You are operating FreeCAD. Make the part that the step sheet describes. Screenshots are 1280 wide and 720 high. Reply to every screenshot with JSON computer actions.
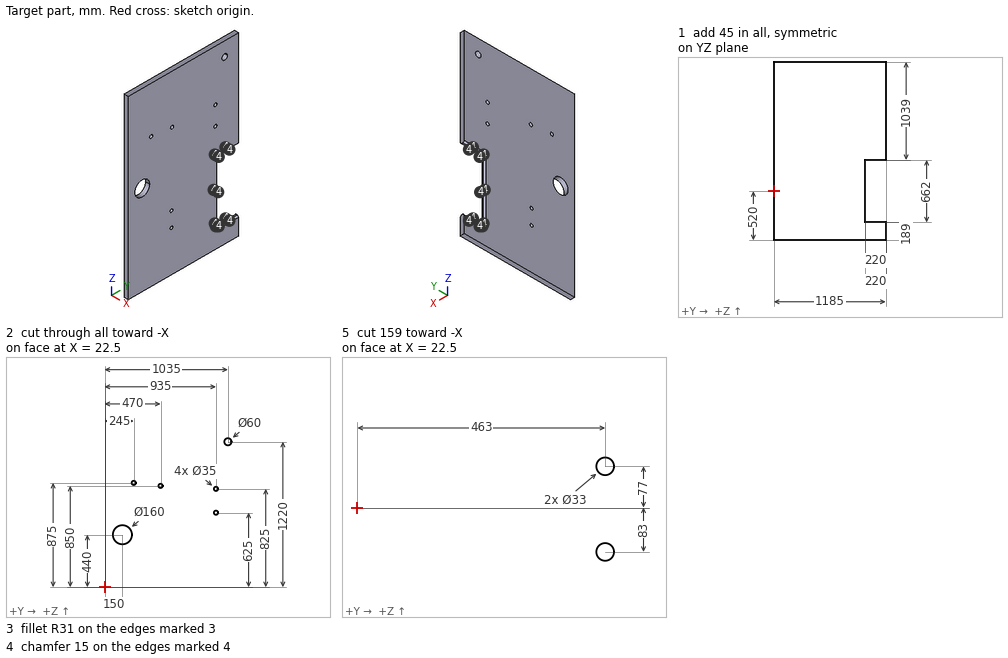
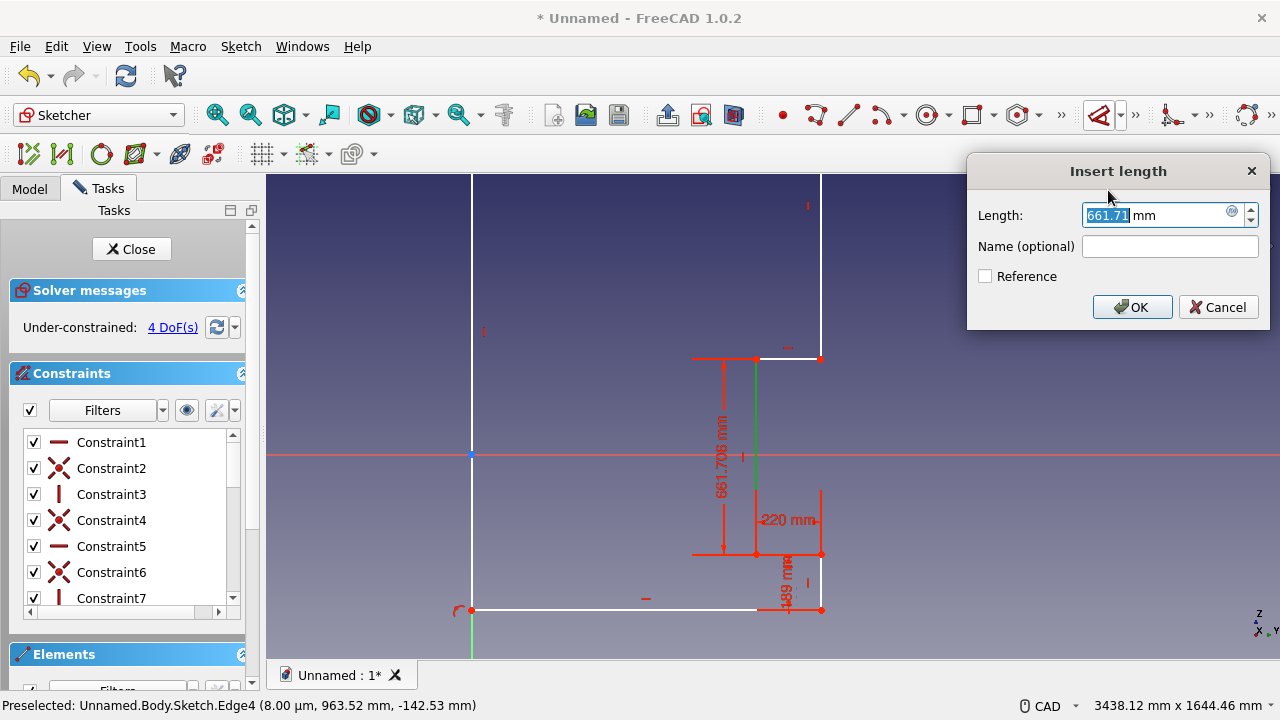
{"action": "type", "text": "662"}
{"action": "key", "text": "Return"}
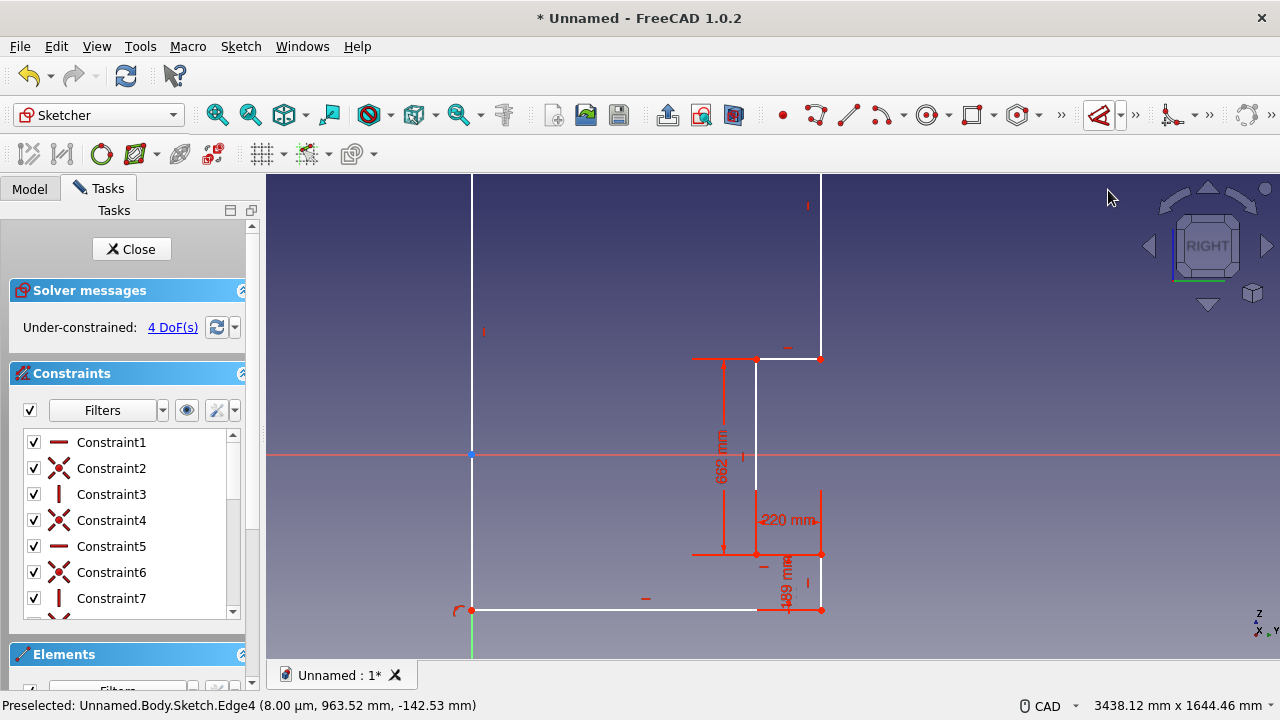
{"action": "left_click", "coordinate": [776, 359]}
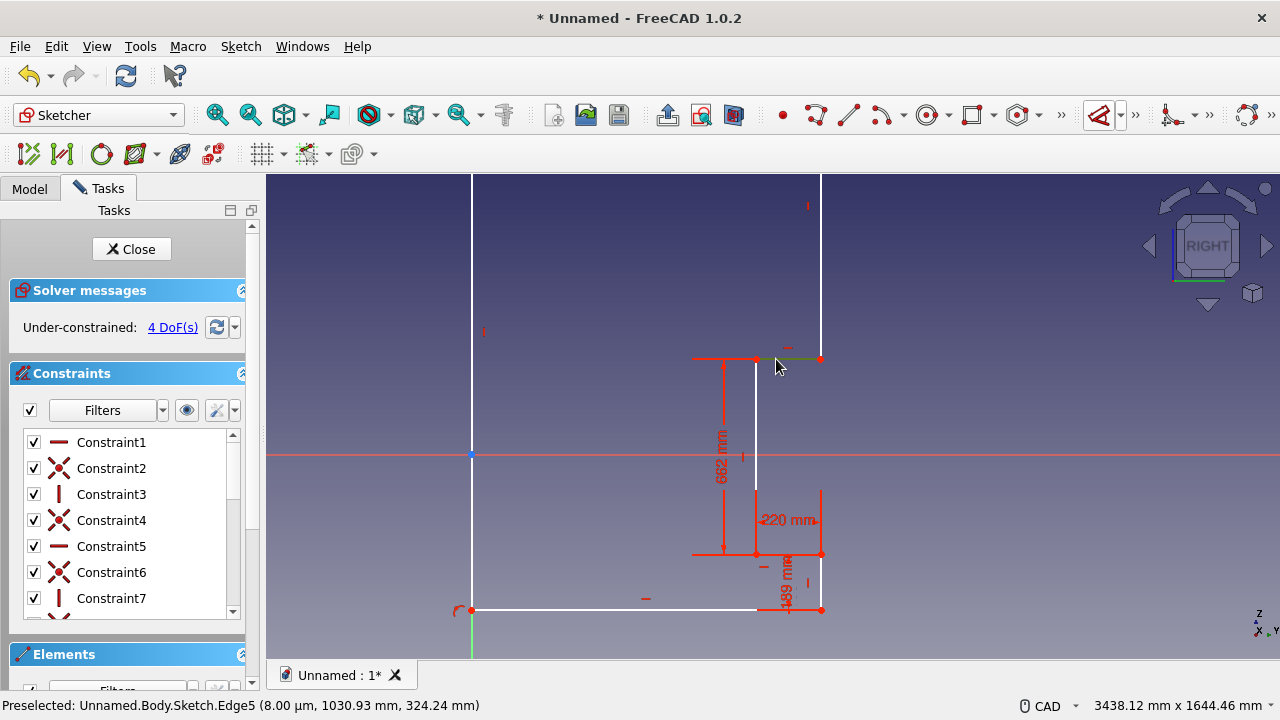
{"action": "key", "text": "l"}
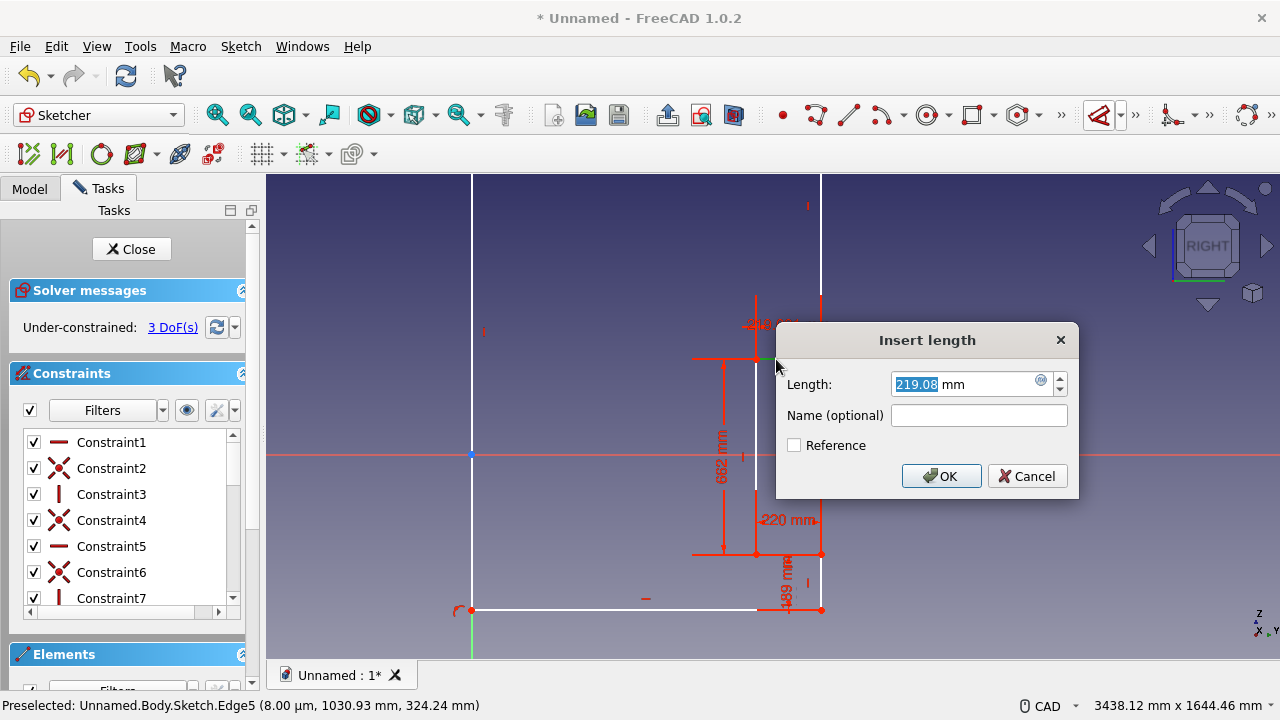
{"action": "type", "text": "220"}
{"action": "key", "text": "Return"}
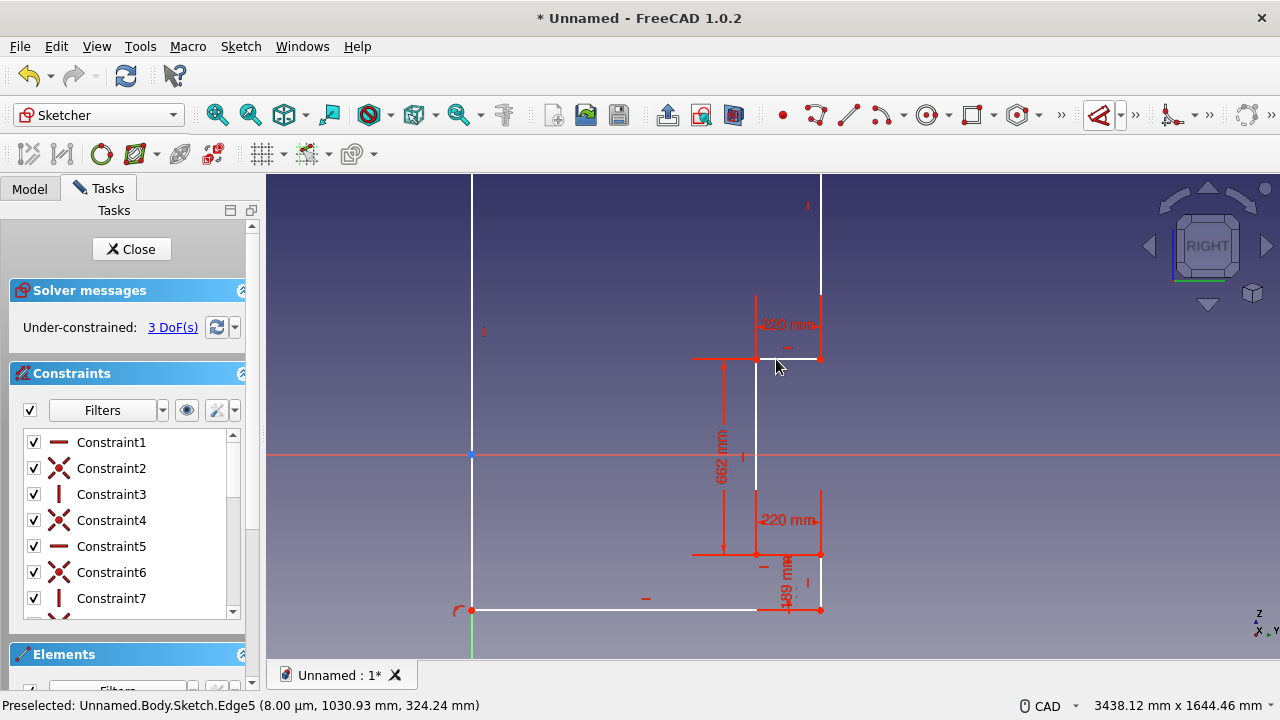
{"action": "left_click", "coordinate": [577, 610]}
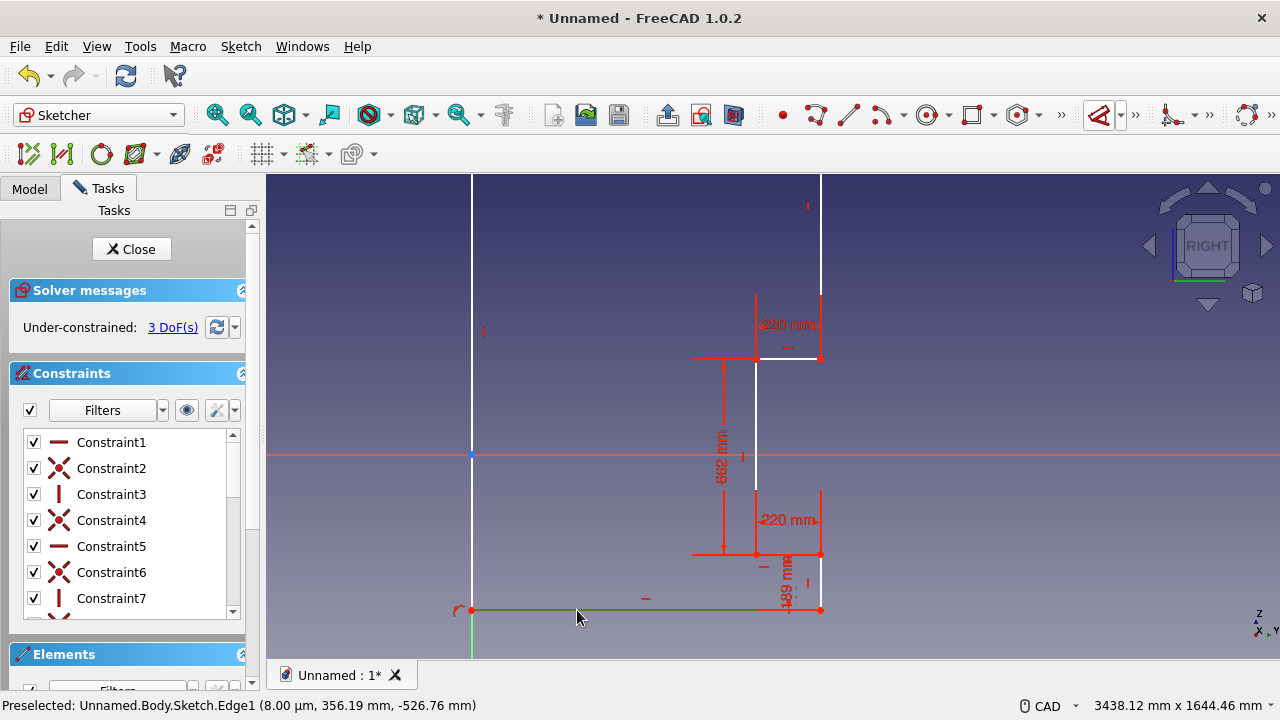
{"action": "left_click", "coordinate": [1120, 116]}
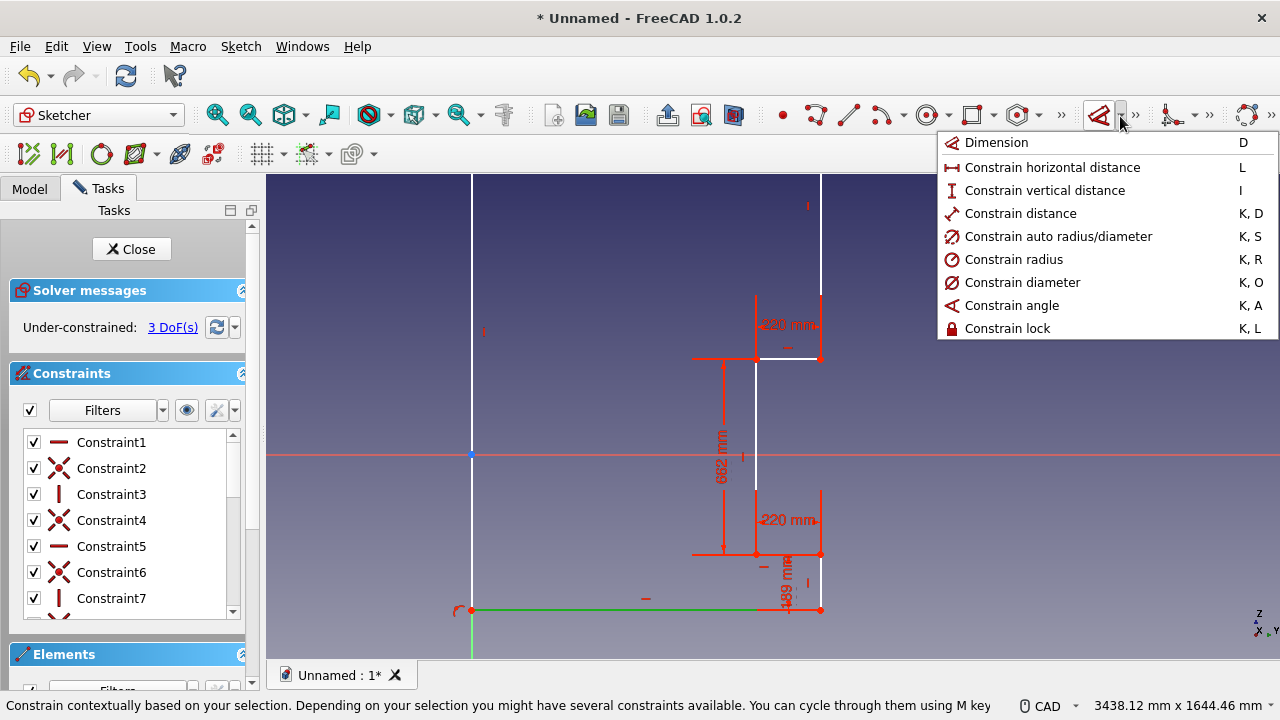
{"action": "left_click", "coordinate": [1108, 168]}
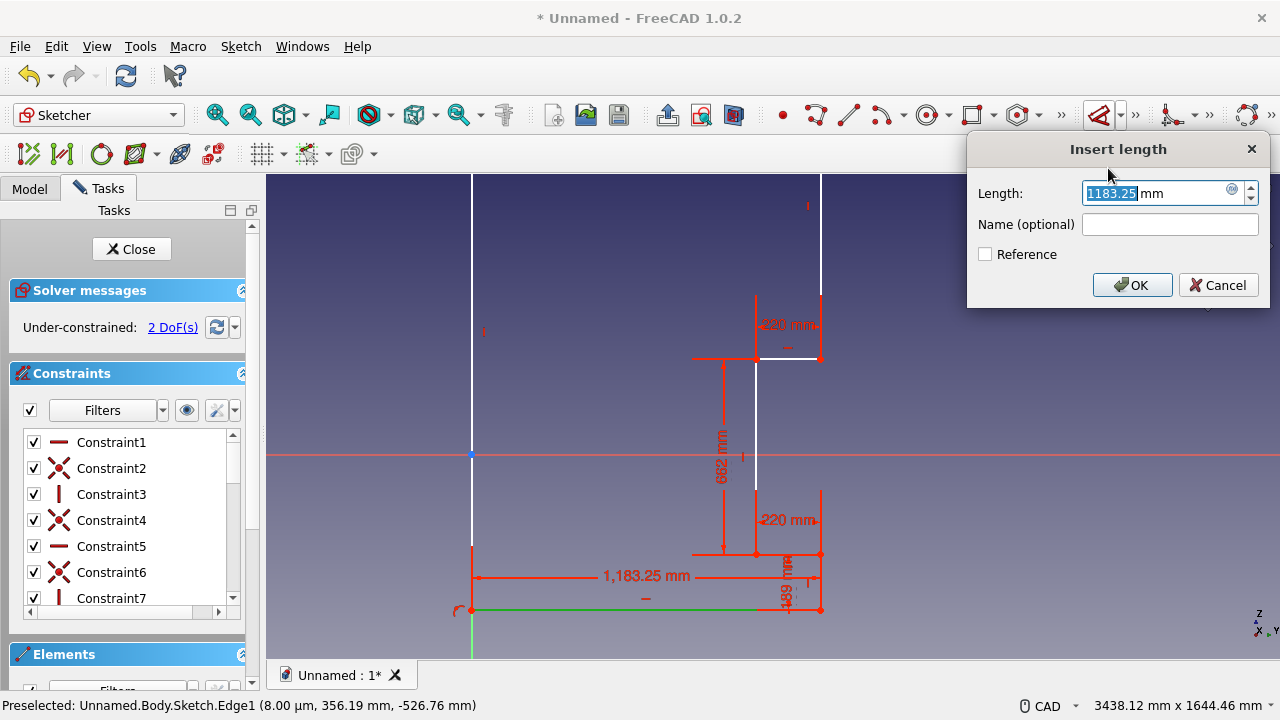
{"action": "type", "text": "1185"}
{"action": "key", "text": "Return"}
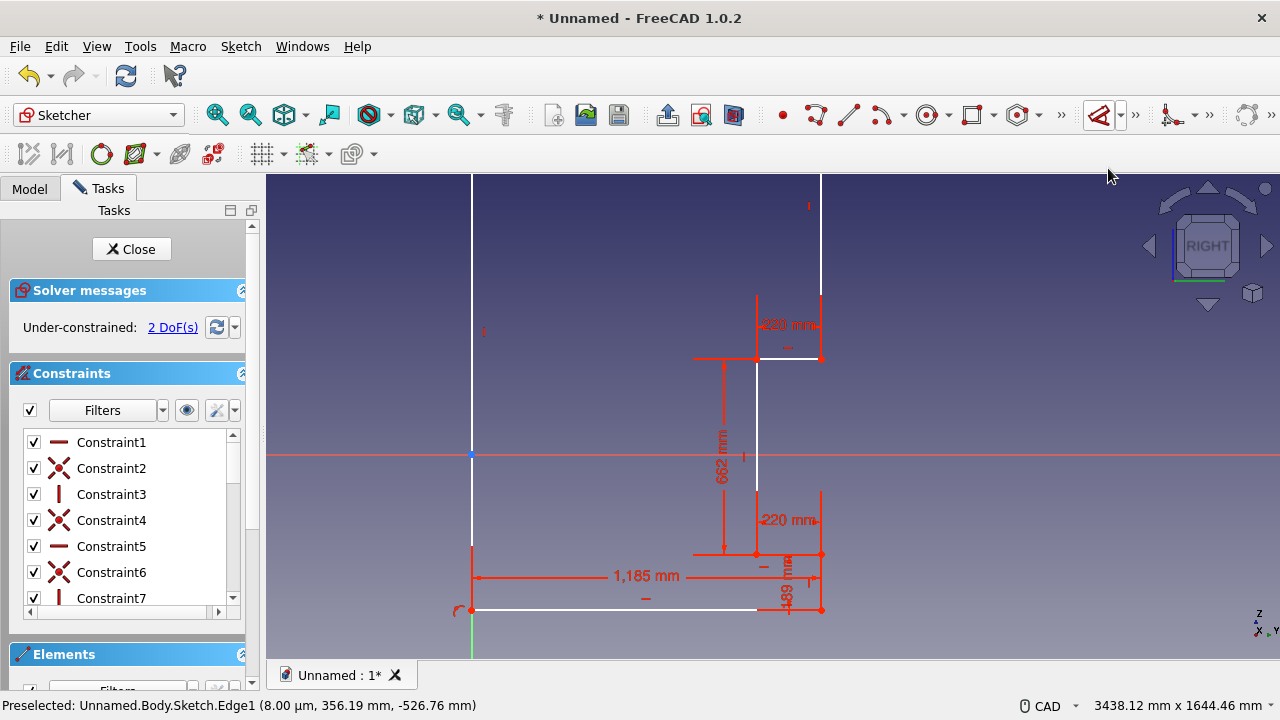
{"action": "left_click", "coordinate": [821, 267]}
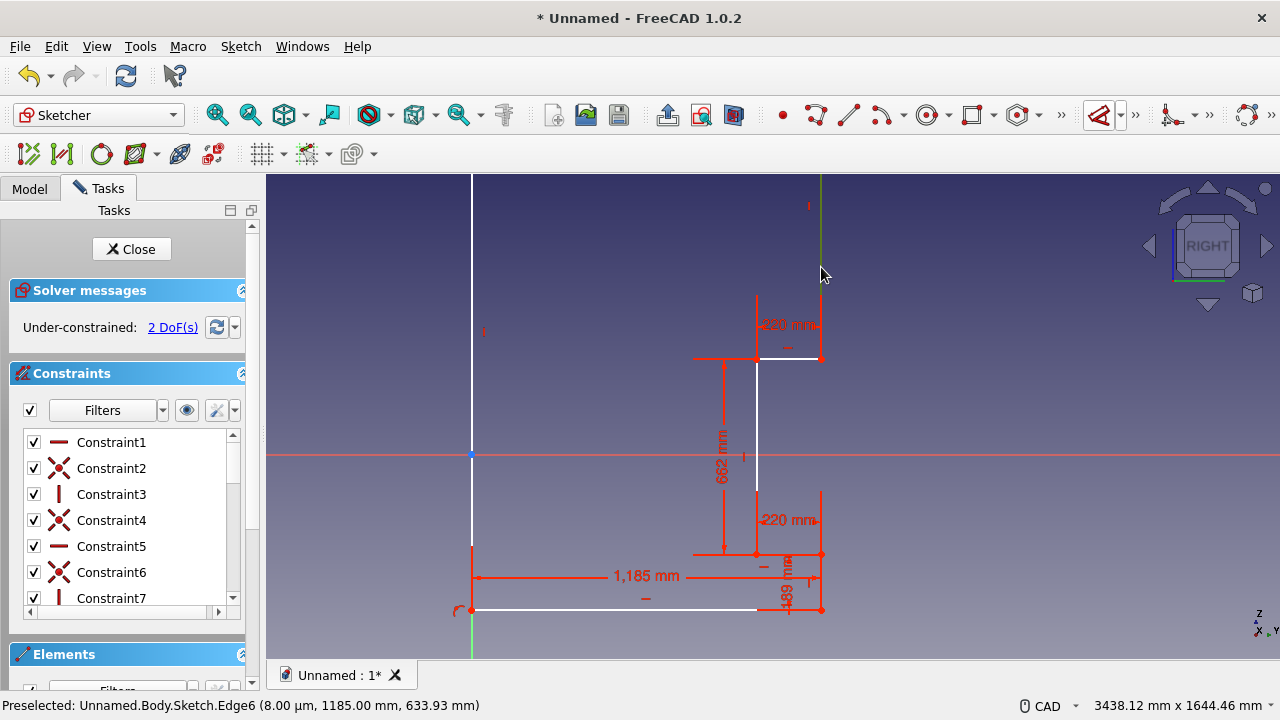
{"action": "left_click", "coordinate": [1120, 116]}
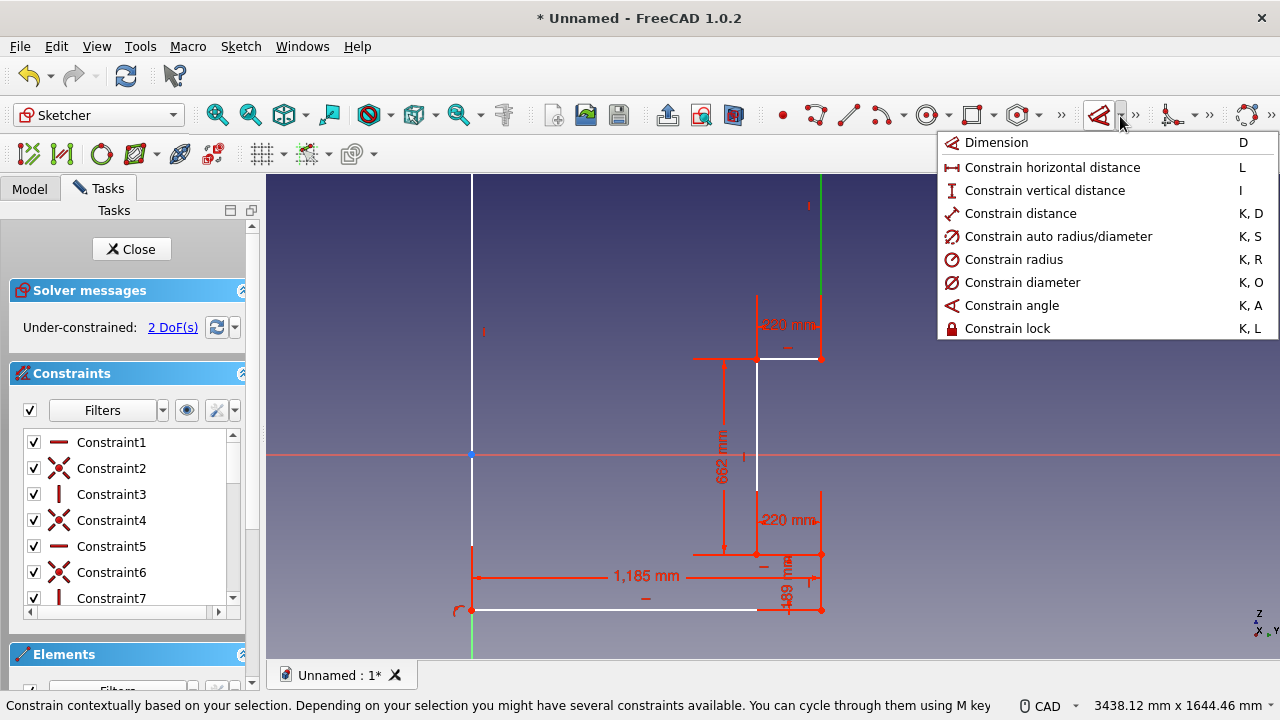
{"action": "left_click", "coordinate": [1108, 190]}